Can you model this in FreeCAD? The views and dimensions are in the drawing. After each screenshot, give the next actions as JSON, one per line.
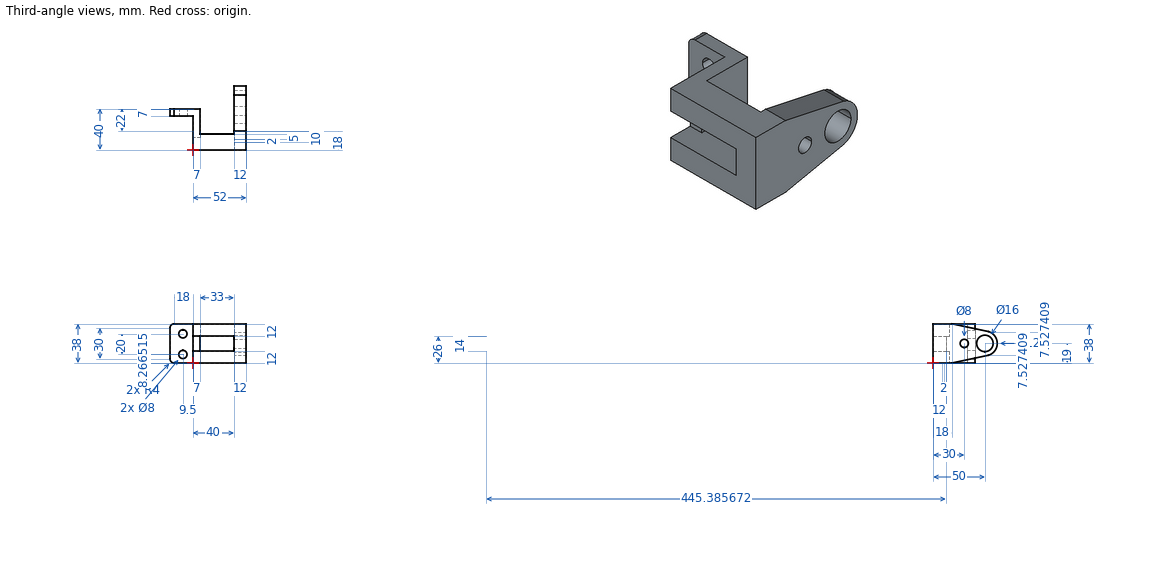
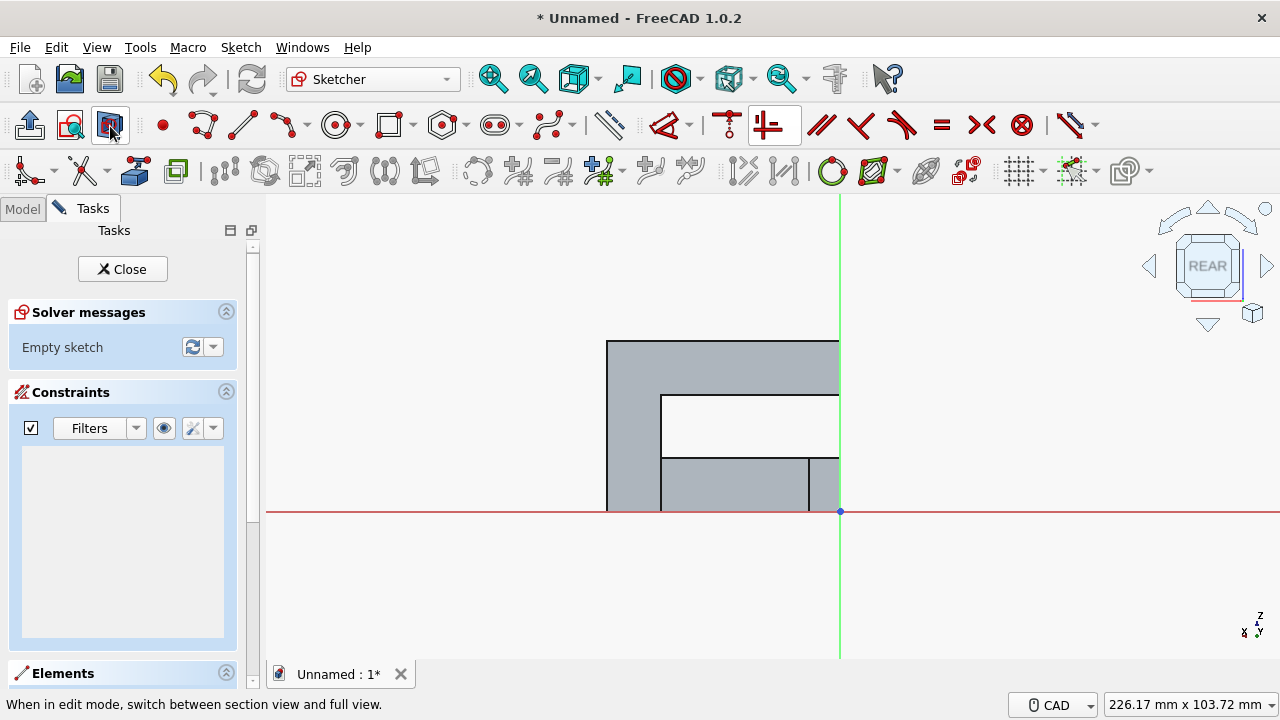
{"action": "scroll", "coordinate": [770, 510], "scroll_direction": "up", "scroll_amount": 6}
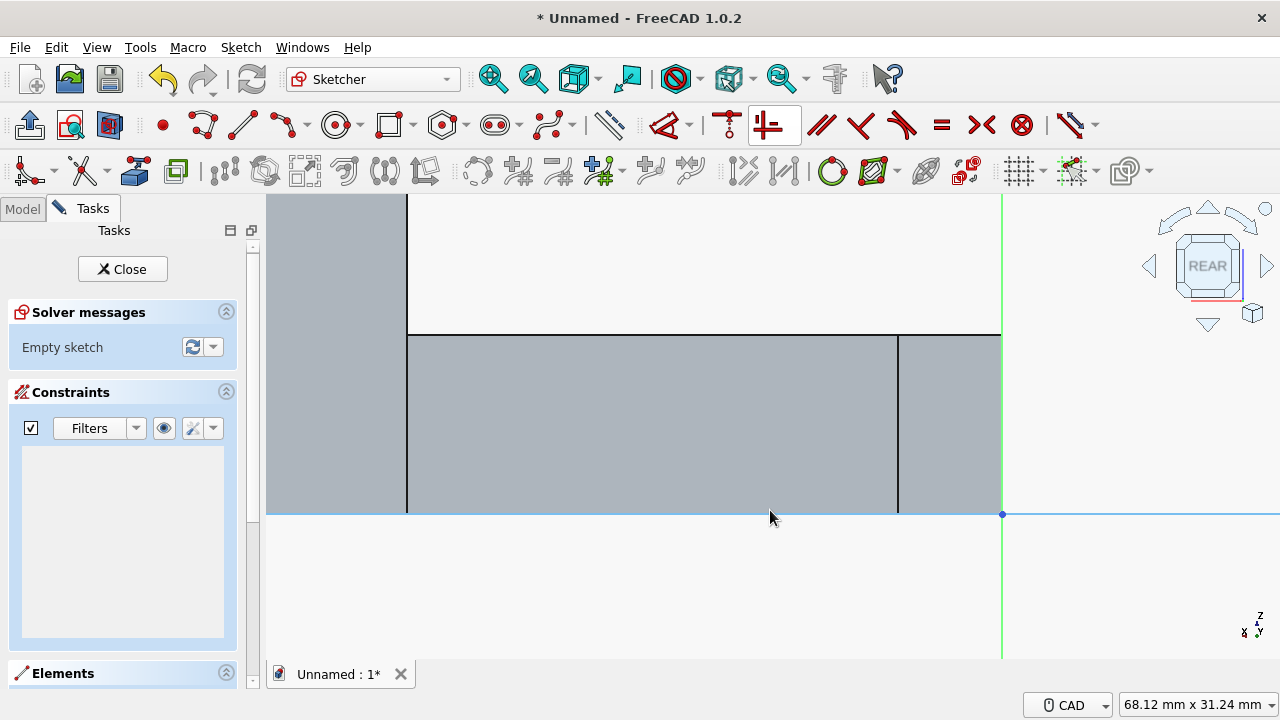
{"action": "left_click", "coordinate": [390, 126]}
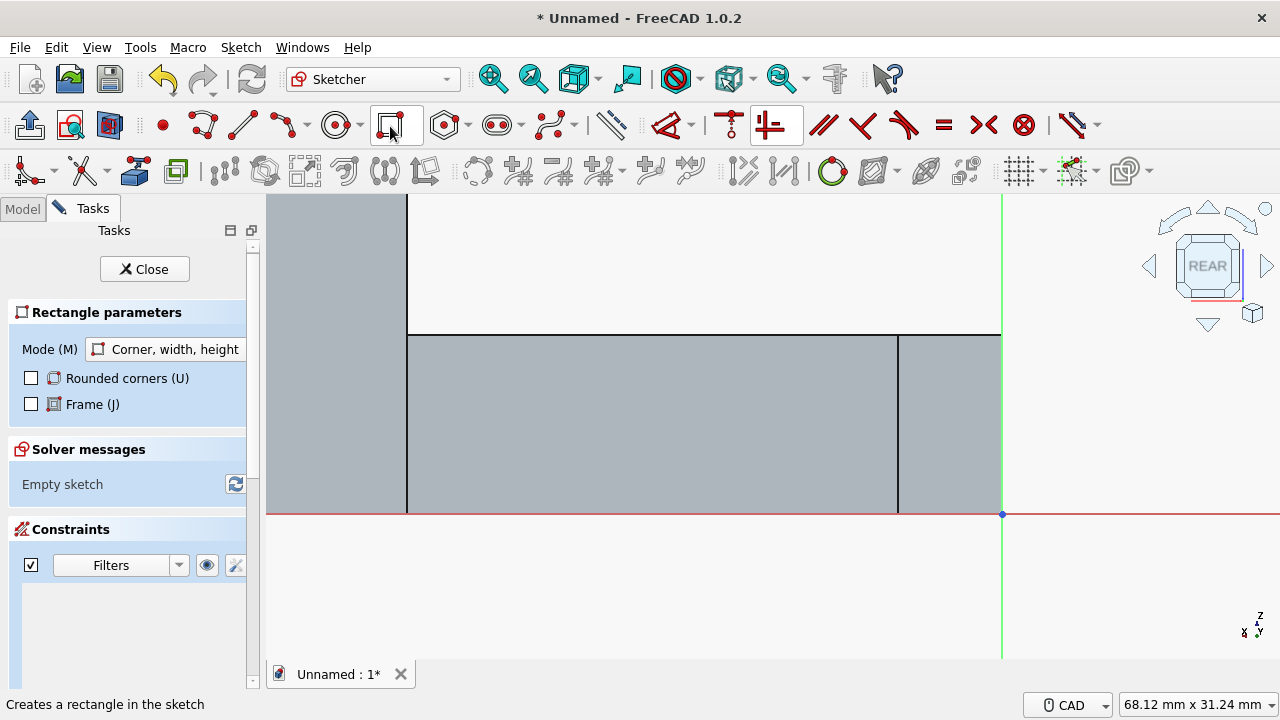
{"action": "left_click", "coordinate": [407, 335]}
{"action": "left_click", "coordinate": [898, 514]}
{"action": "key", "text": "Escape"}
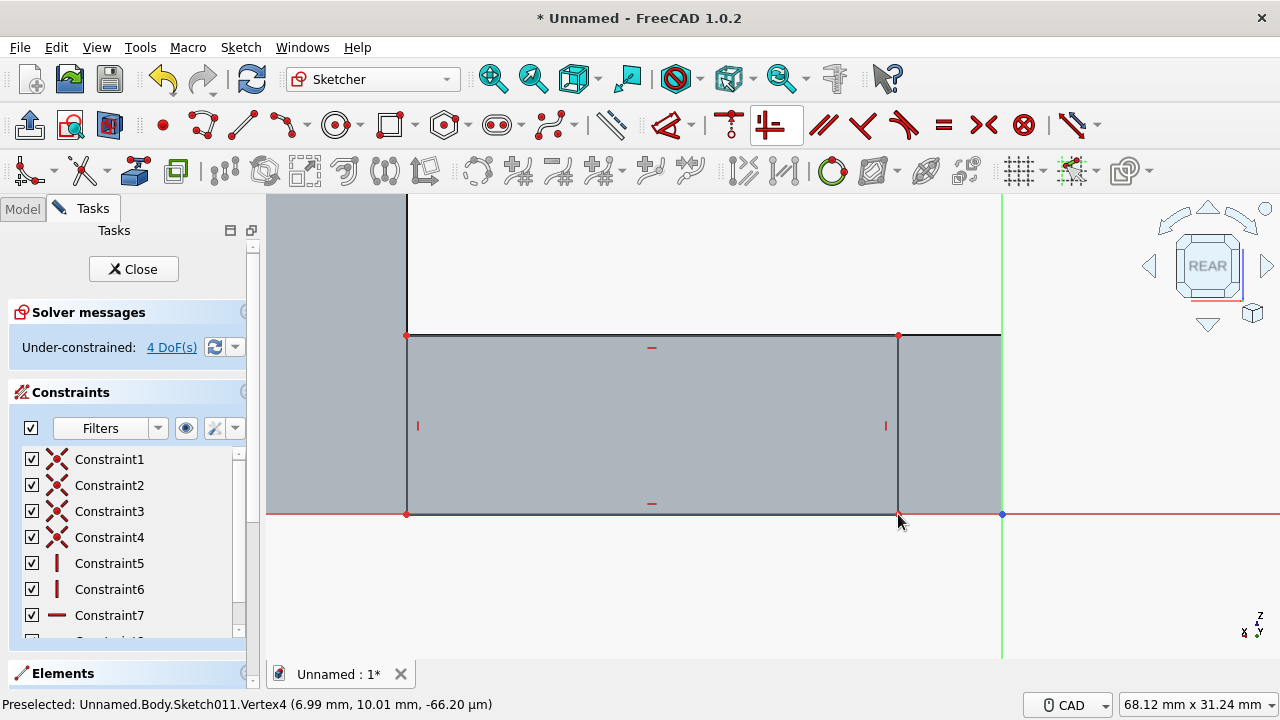
{"action": "left_click", "coordinate": [407, 515]}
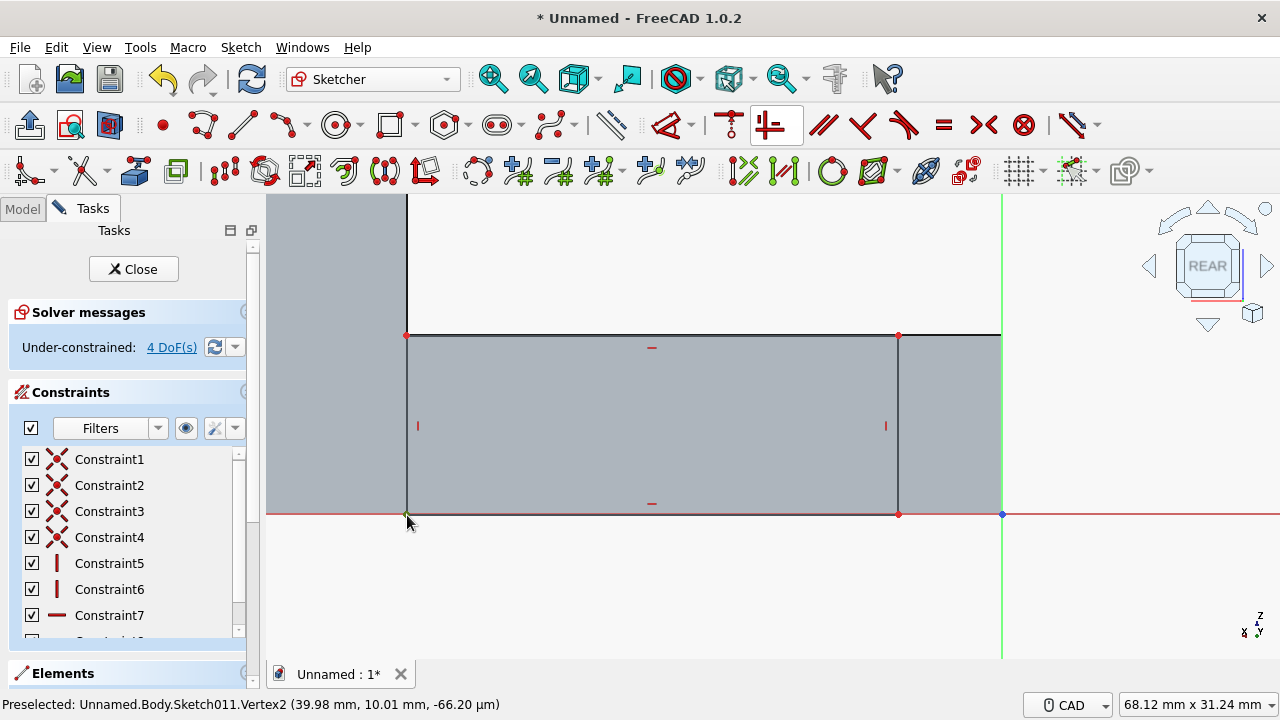
{"action": "left_click", "coordinate": [353, 514]}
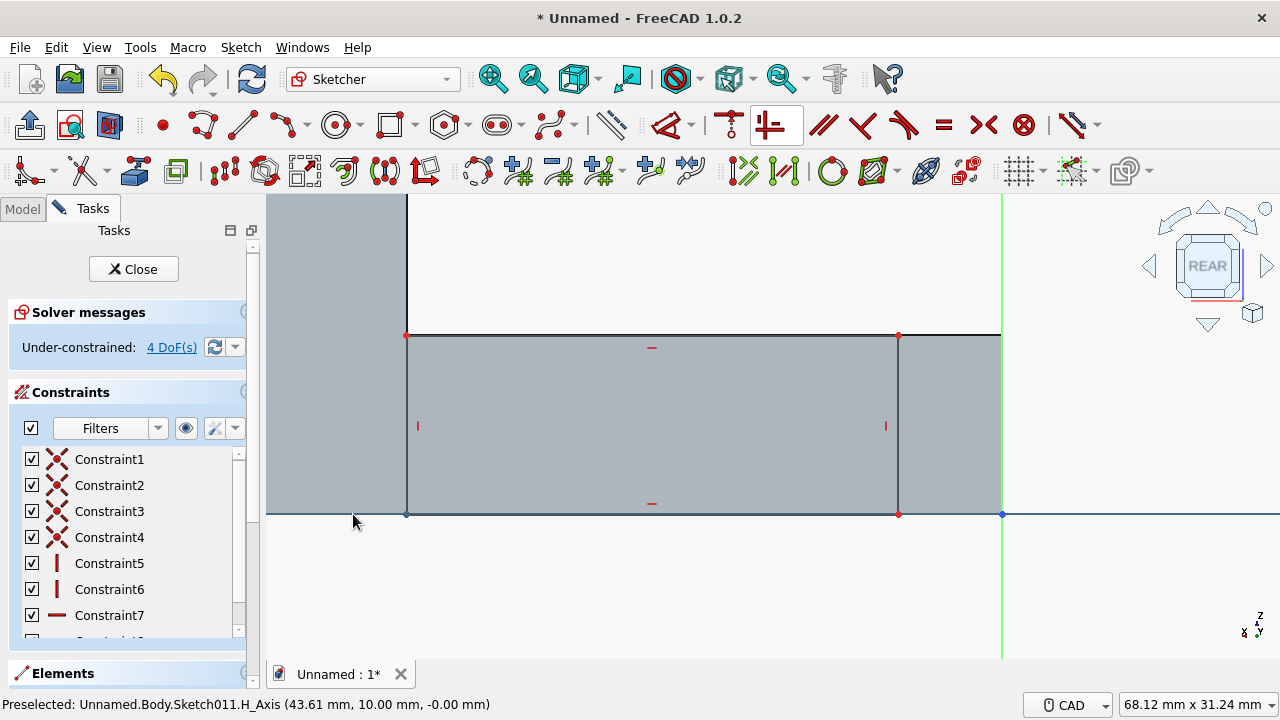
{"action": "left_click", "coordinate": [730, 126]}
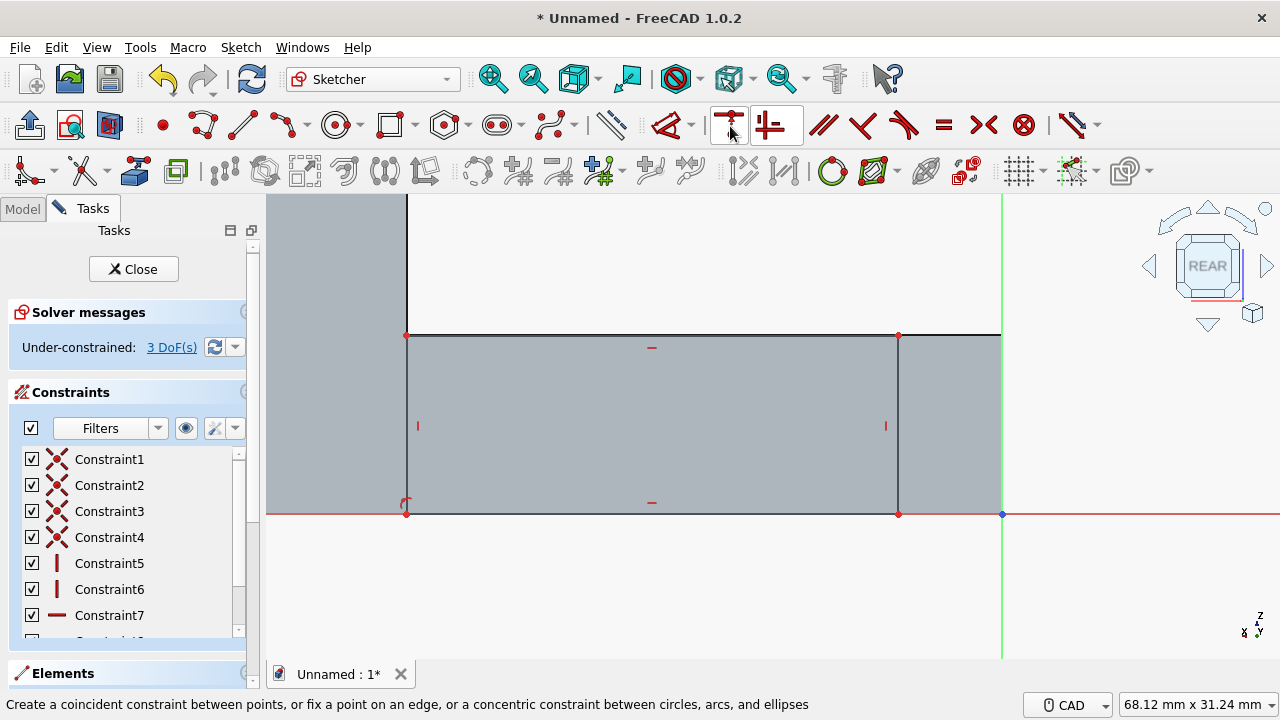
{"action": "left_click", "coordinate": [666, 126]}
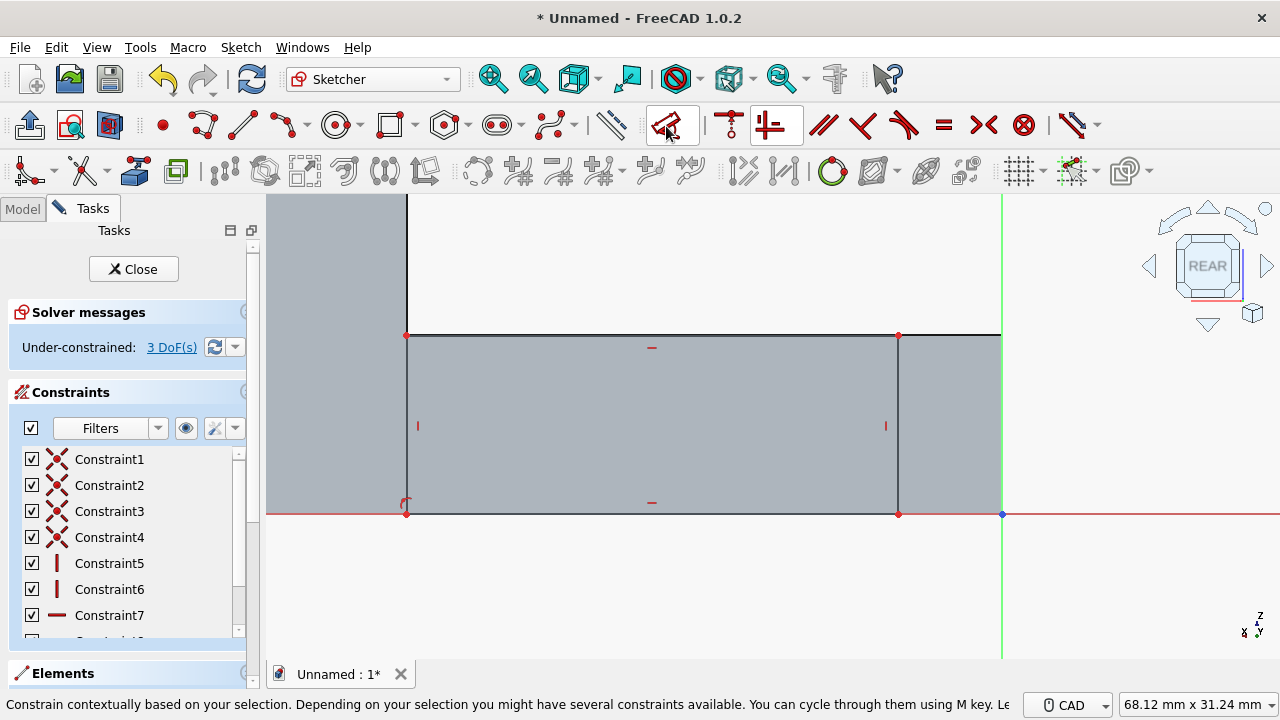
{"action": "left_click", "coordinate": [407, 389]}
{"action": "left_click", "coordinate": [373, 425]}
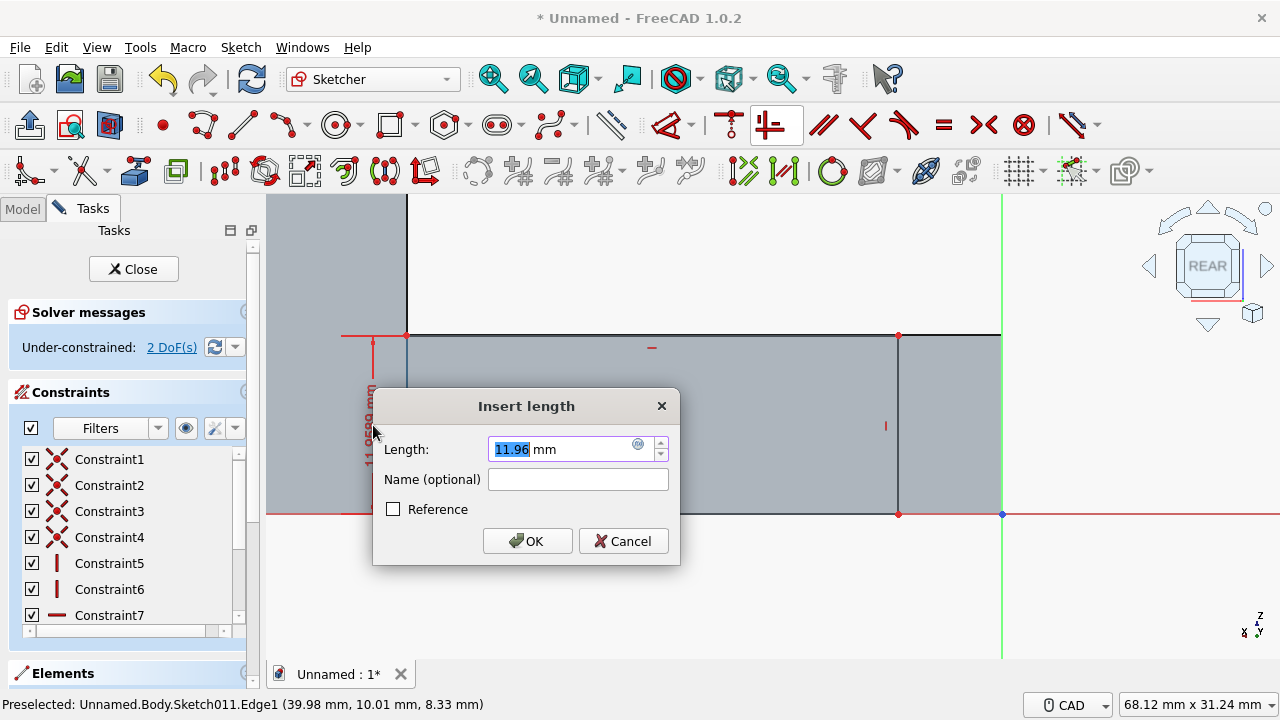
{"action": "type", "text": "12"}
{"action": "key", "text": "Return"}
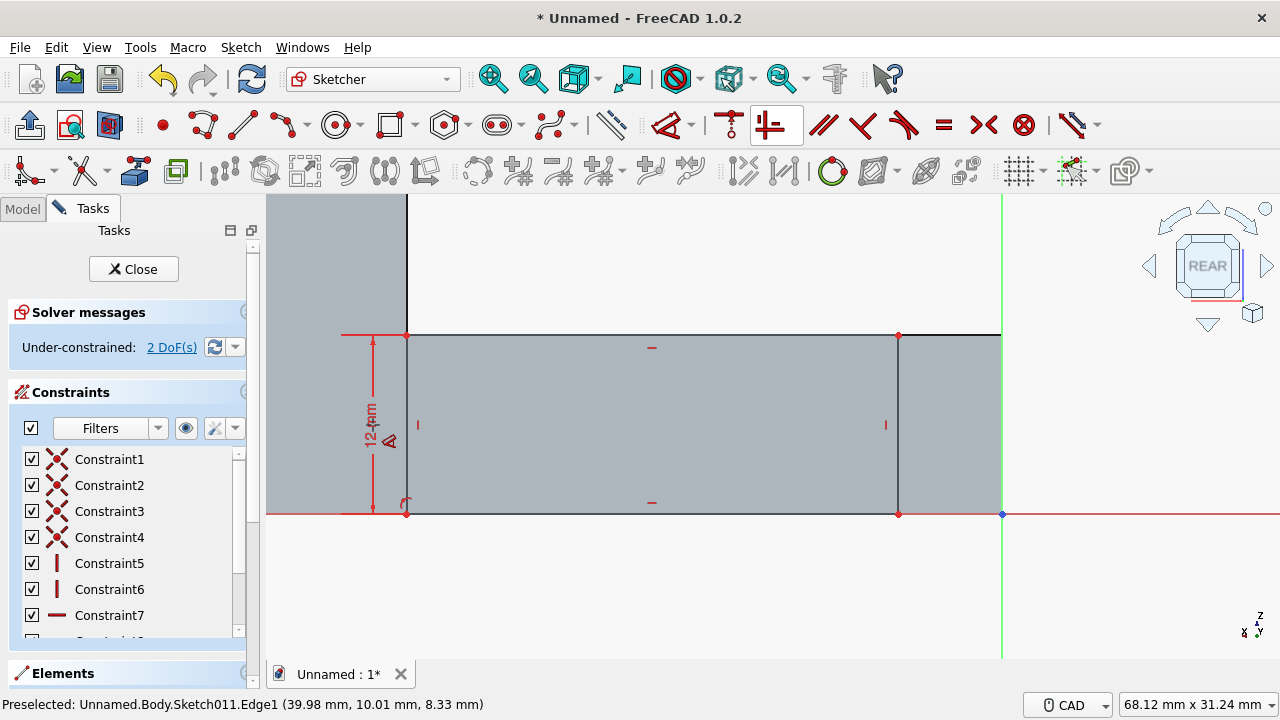
{"action": "left_click", "coordinate": [554, 514]}
{"action": "left_click", "coordinate": [652, 548]}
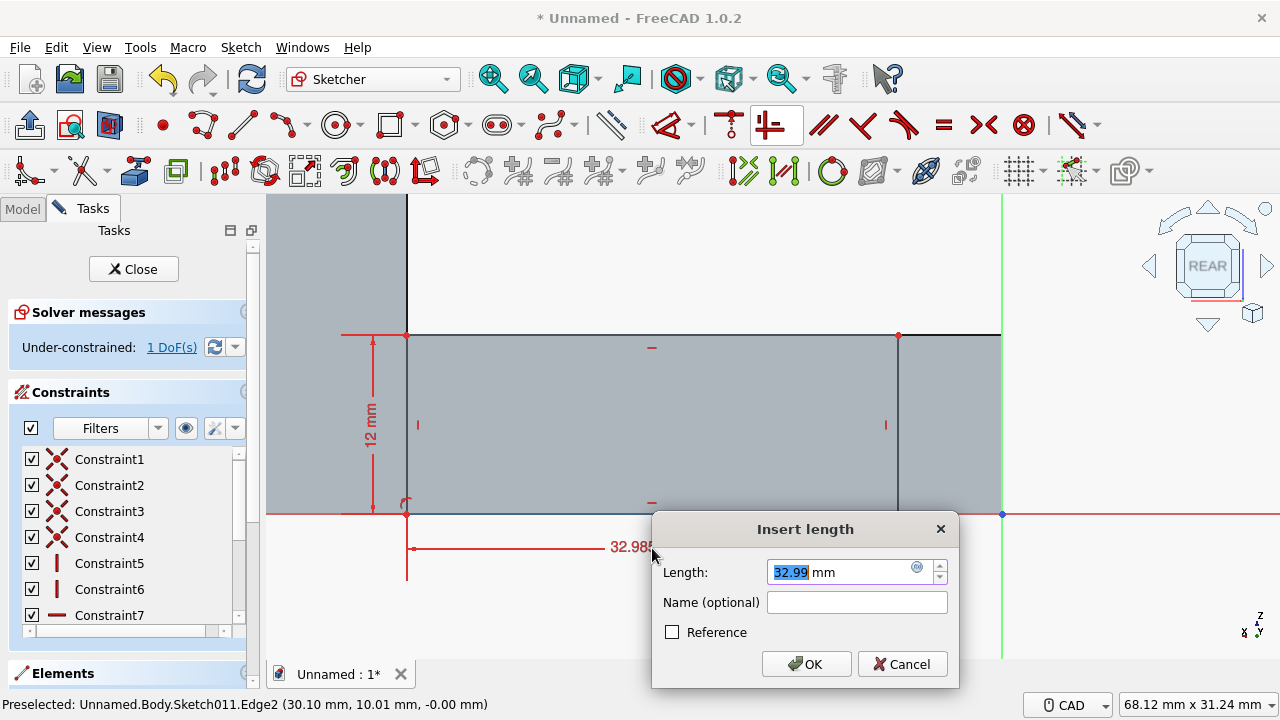
{"action": "type", "text": "33"}
{"action": "key", "text": "Return"}